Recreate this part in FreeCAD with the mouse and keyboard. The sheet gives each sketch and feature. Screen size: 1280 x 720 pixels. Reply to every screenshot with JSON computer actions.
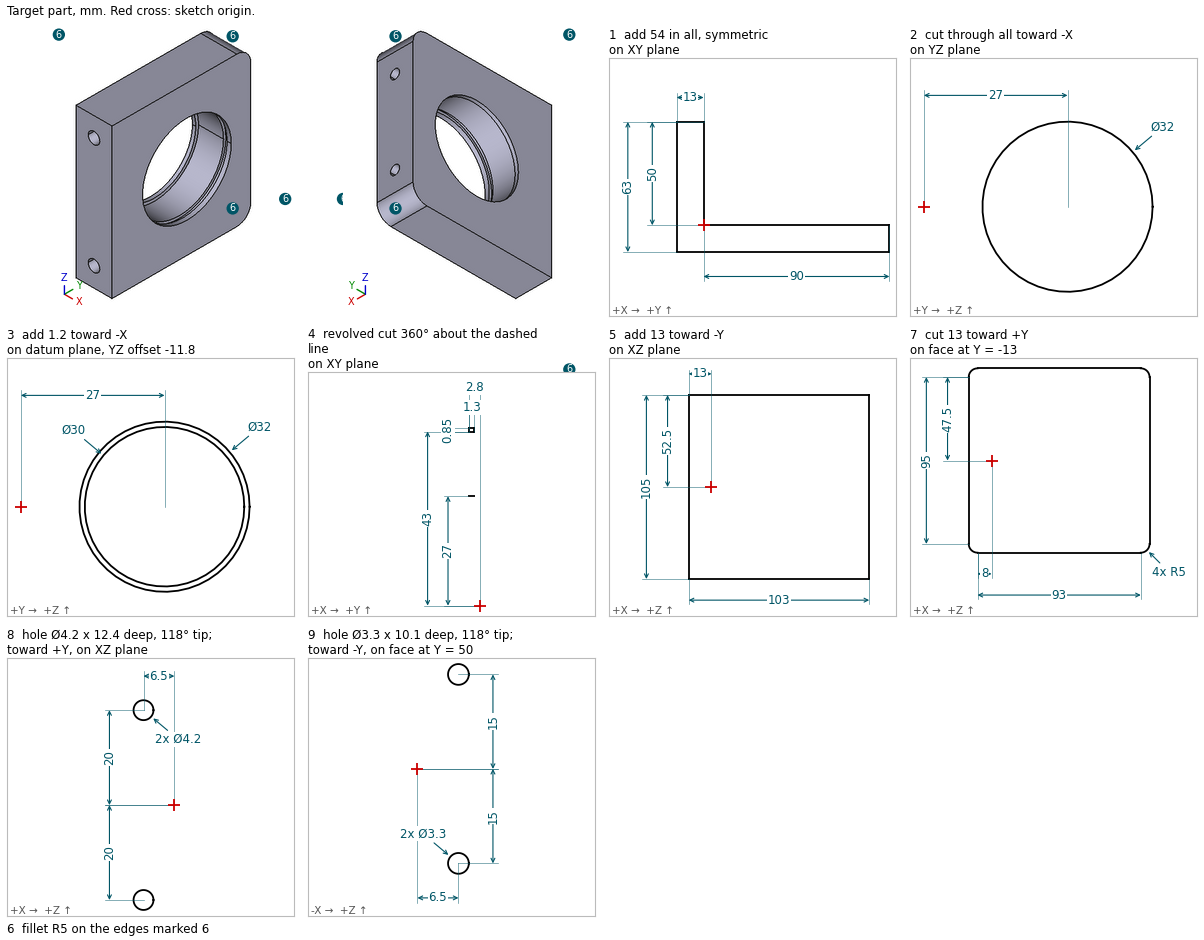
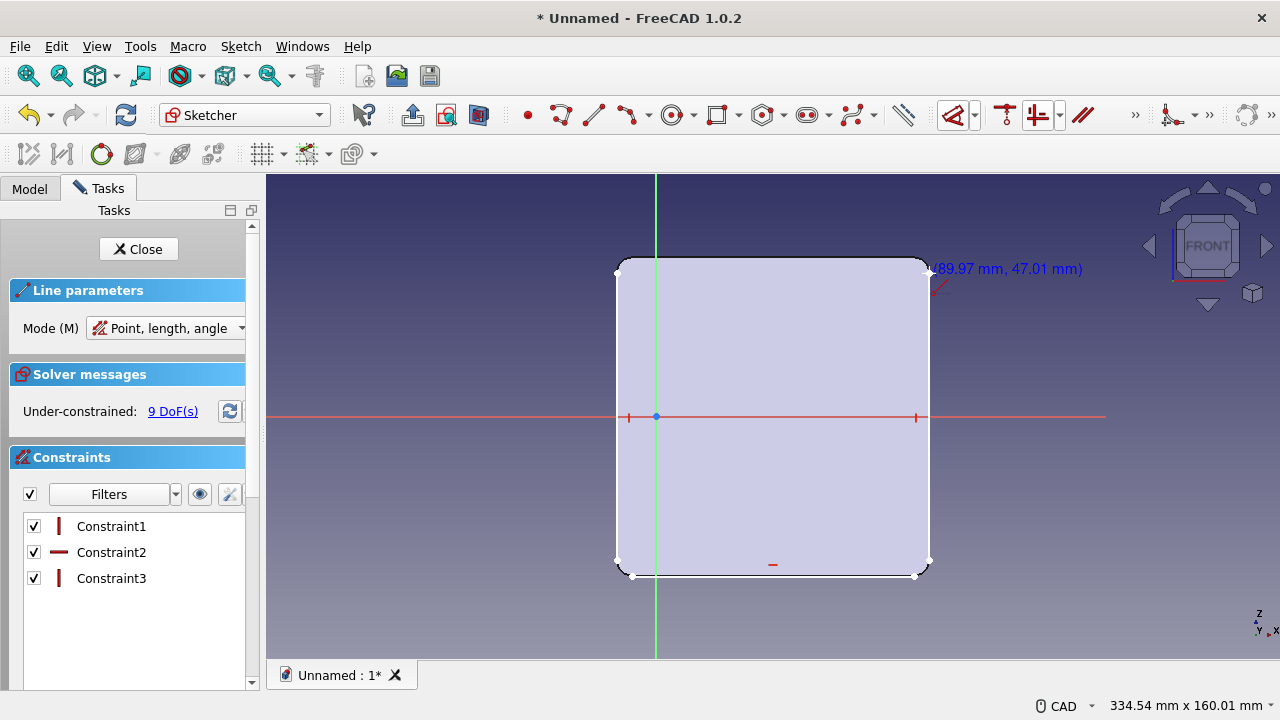
{"action": "left_click", "coordinate": [914, 257]}
{"action": "left_click", "coordinate": [632, 257]}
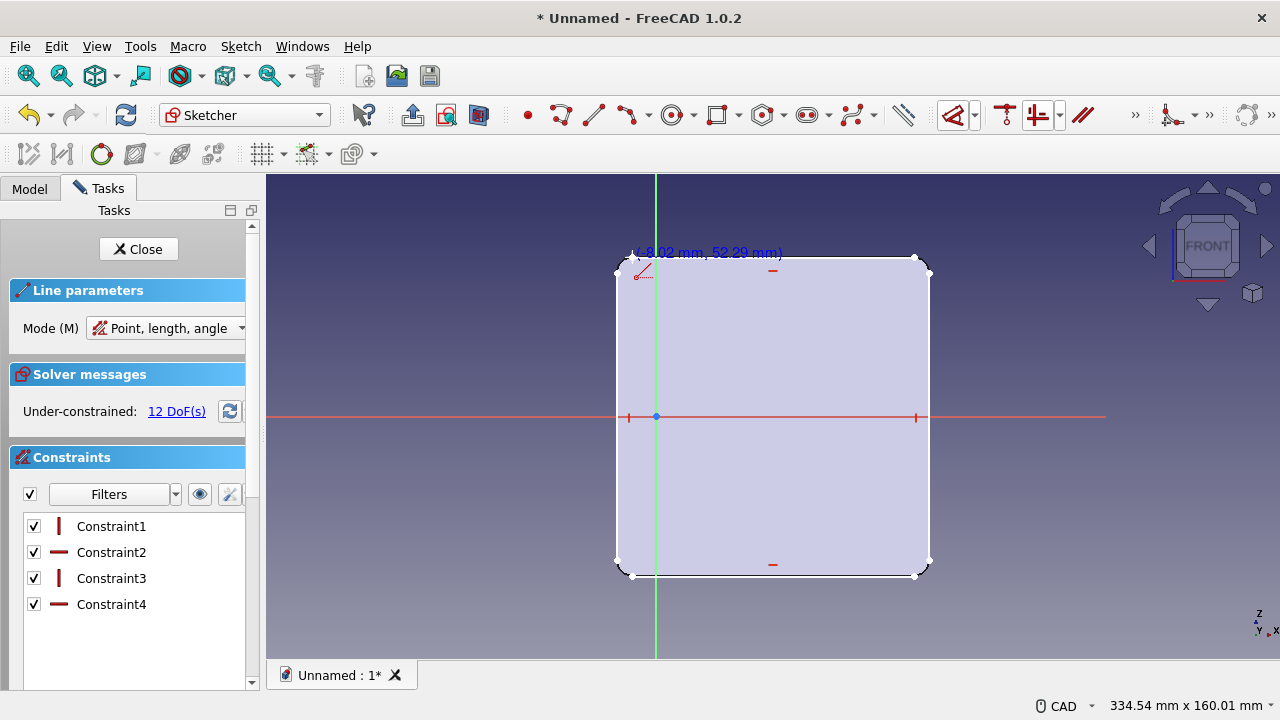
{"action": "left_click", "coordinate": [626, 116]}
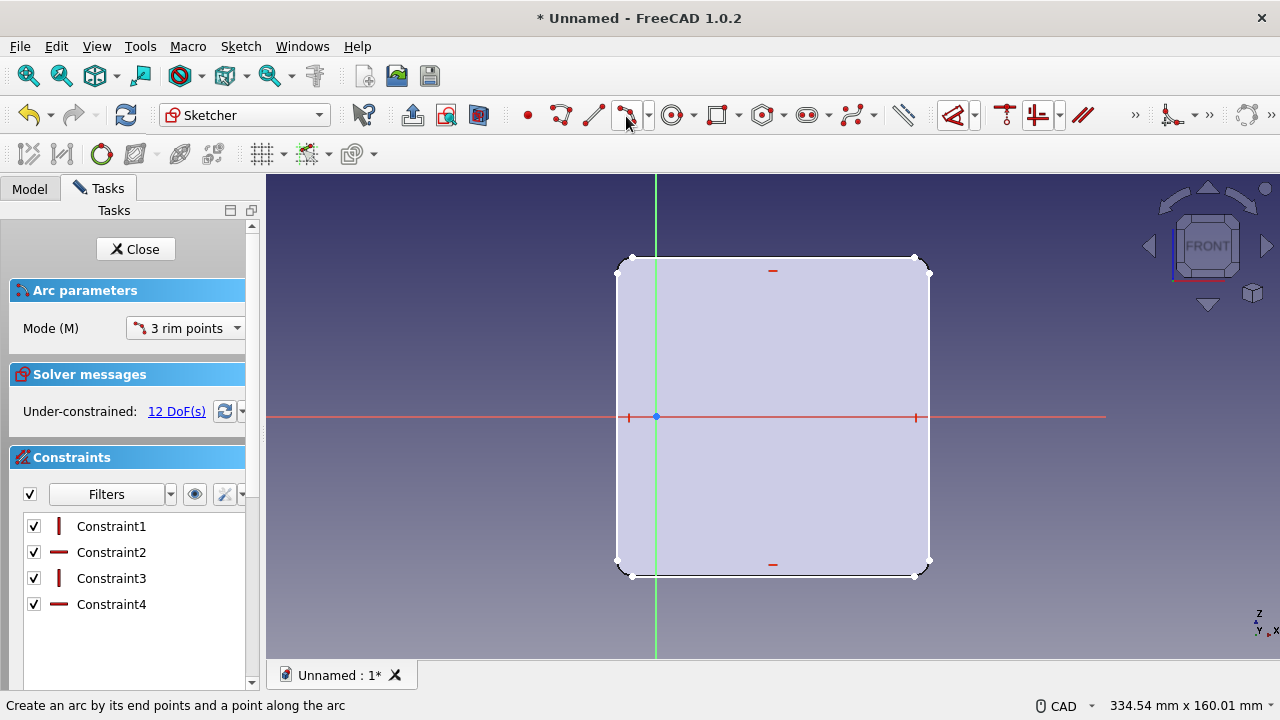
{"action": "left_click", "coordinate": [617, 561]}
{"action": "left_click", "coordinate": [632, 577]}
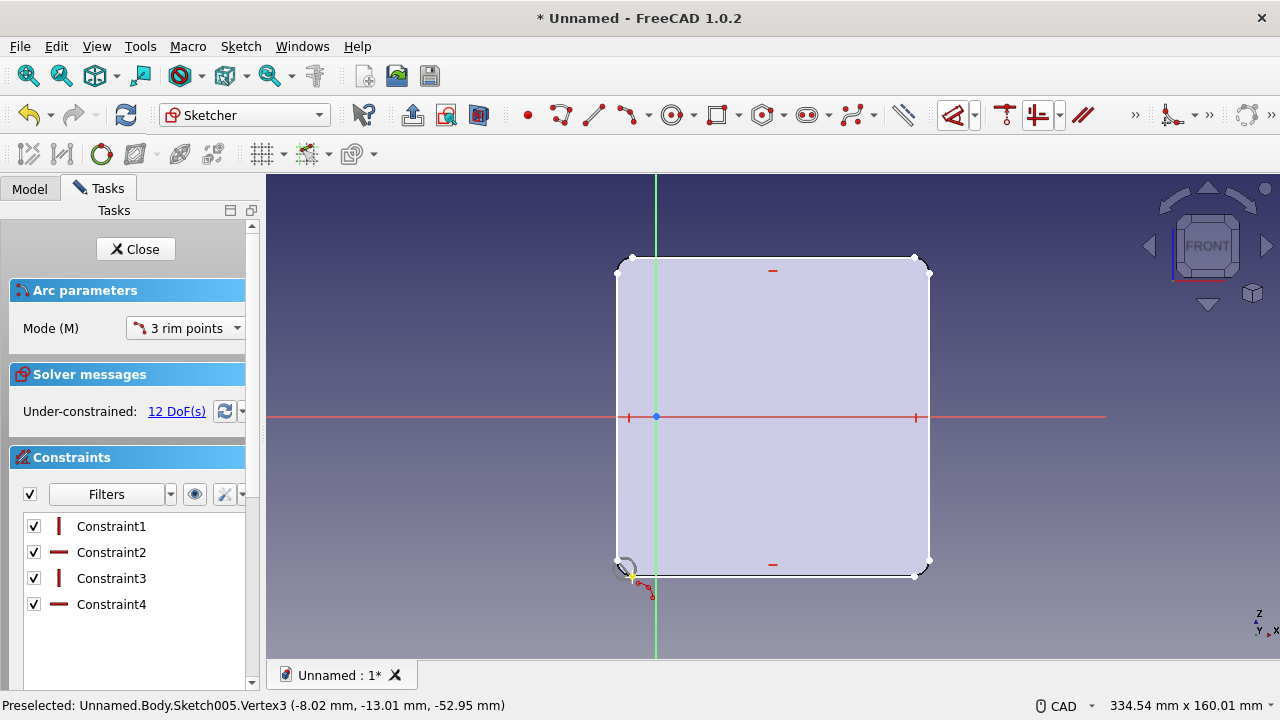
{"action": "scroll", "coordinate": [621, 571], "scroll_direction": "up", "scroll_amount": 7}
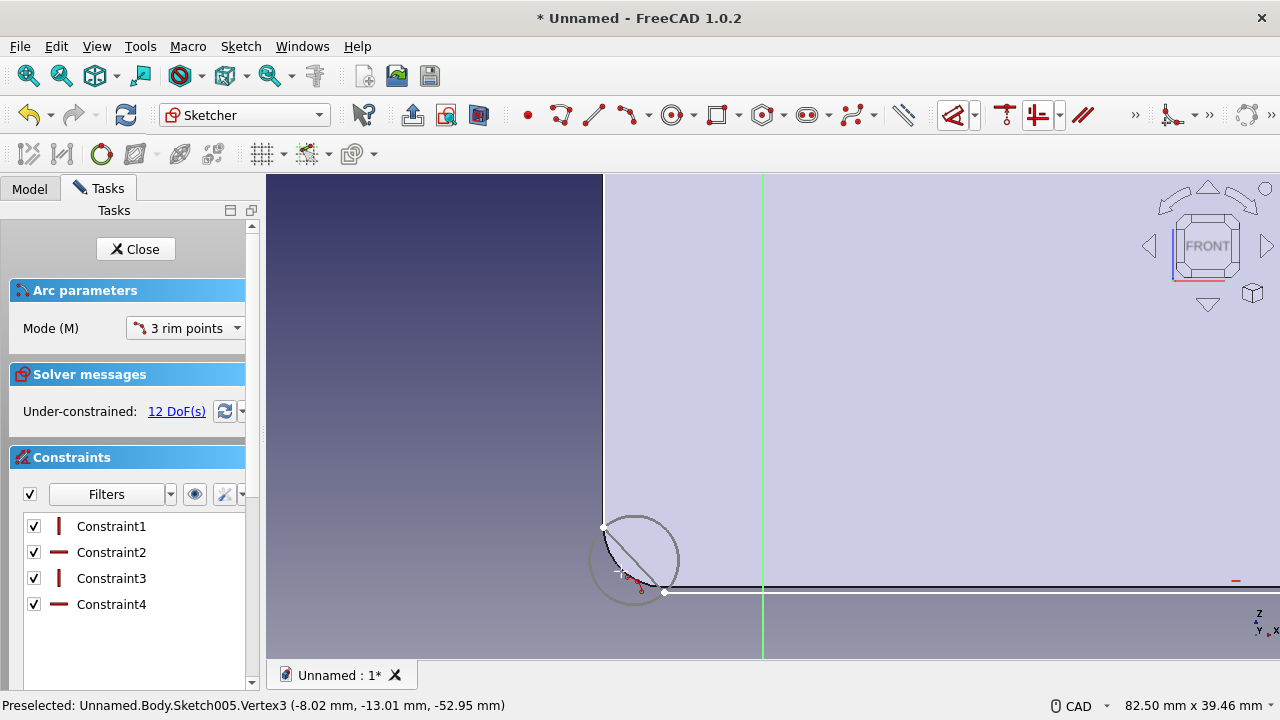
{"action": "left_click", "coordinate": [621, 569]}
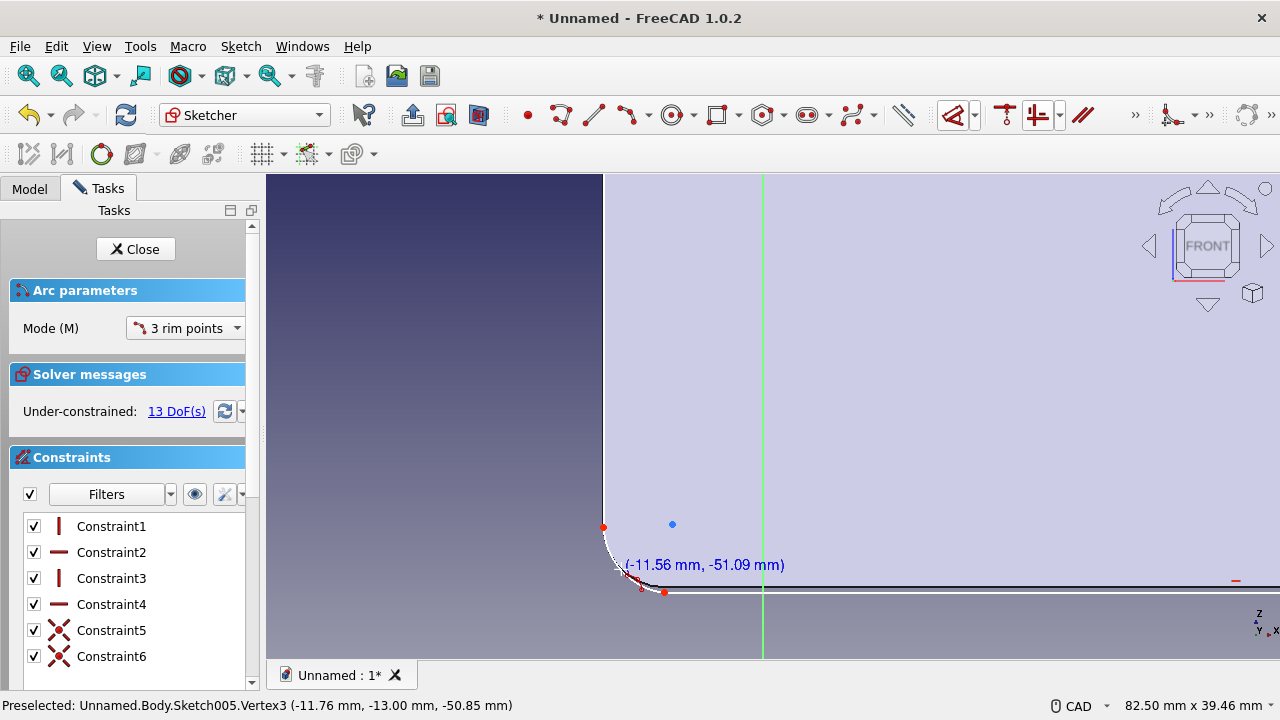
{"action": "scroll", "coordinate": [530, 572], "scroll_direction": "down", "scroll_amount": 7}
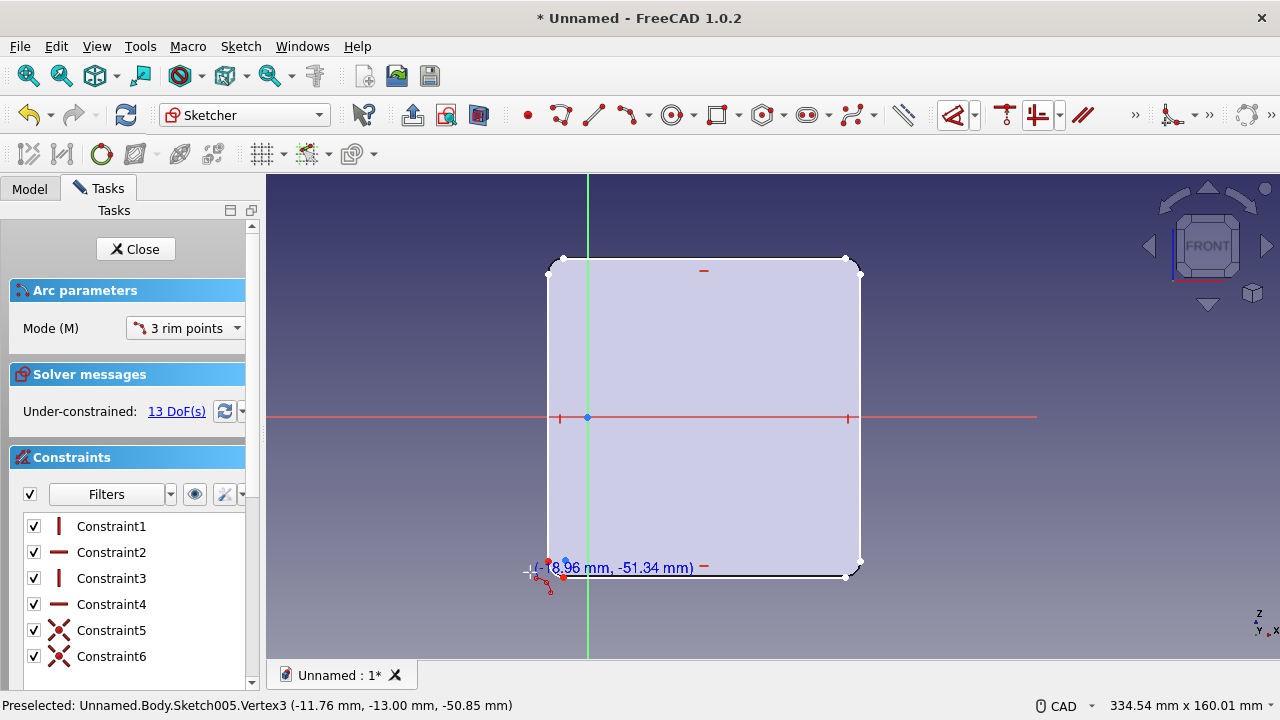
{"action": "left_click", "coordinate": [845, 578]}
{"action": "left_click", "coordinate": [860, 562]}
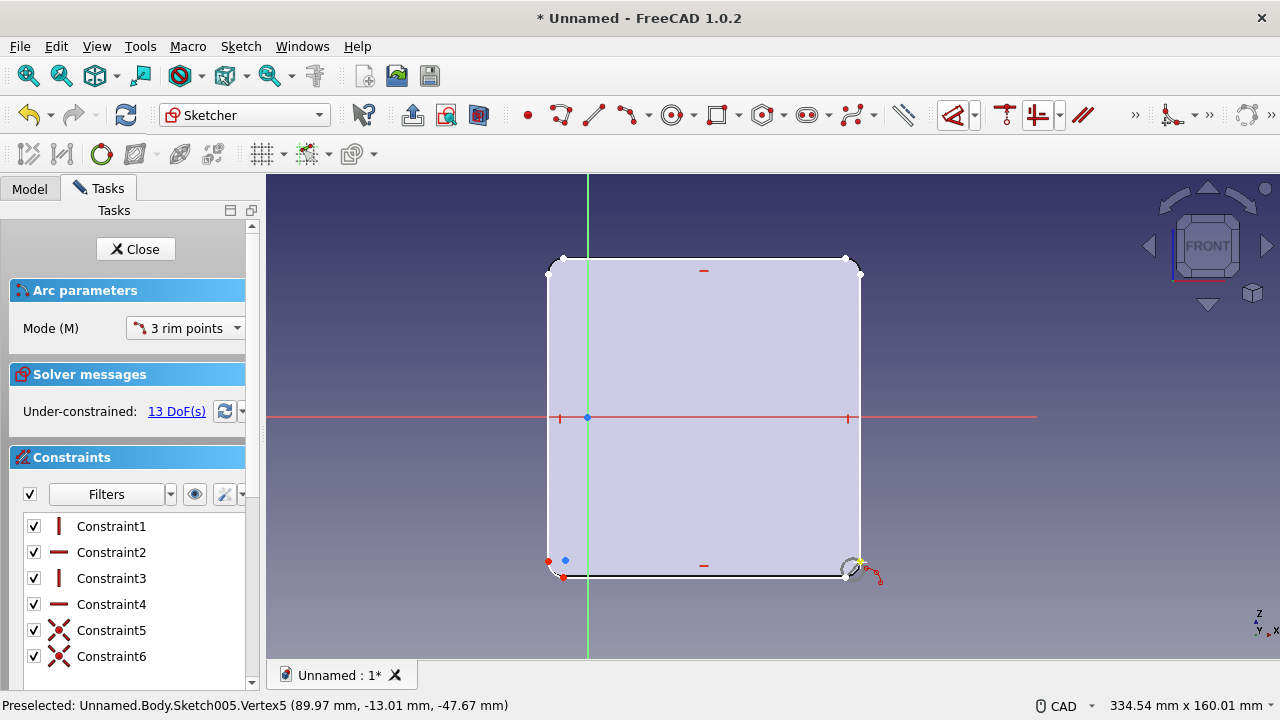
{"action": "scroll", "coordinate": [856, 572], "scroll_direction": "up", "scroll_amount": 7}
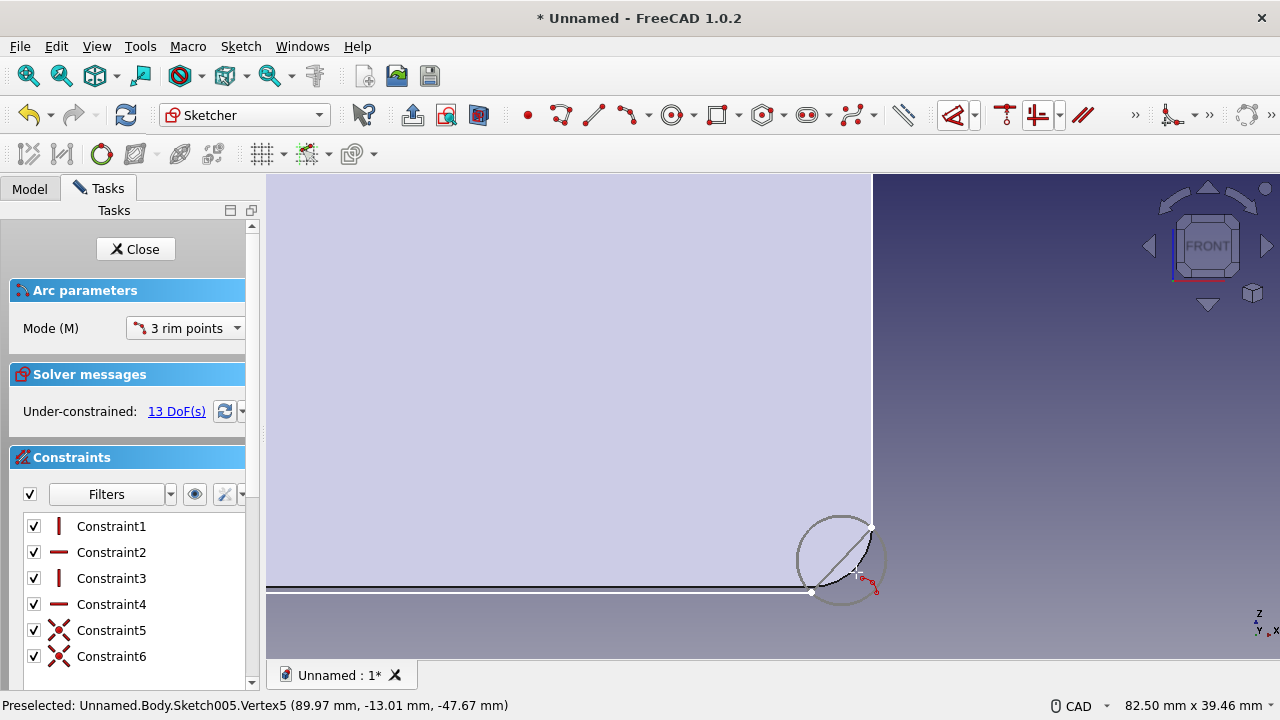
{"action": "left_click", "coordinate": [854, 569]}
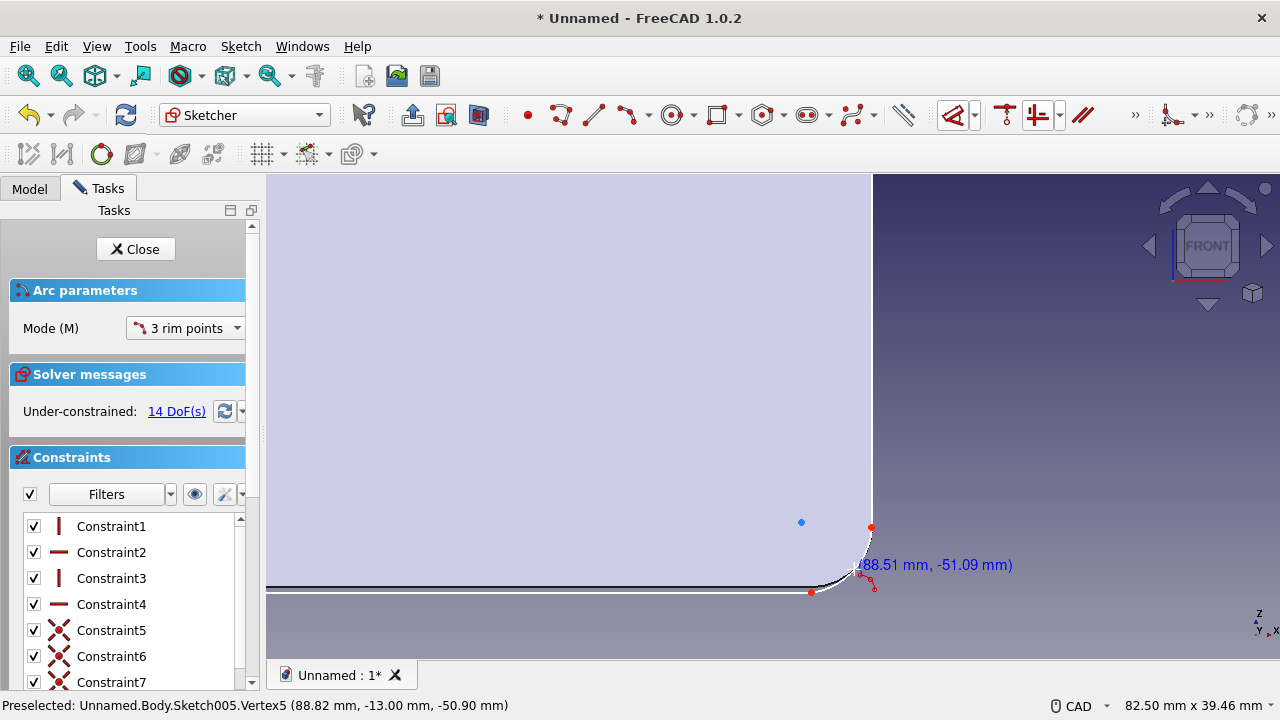
{"action": "scroll", "coordinate": [857, 572], "scroll_direction": "down", "scroll_amount": 7}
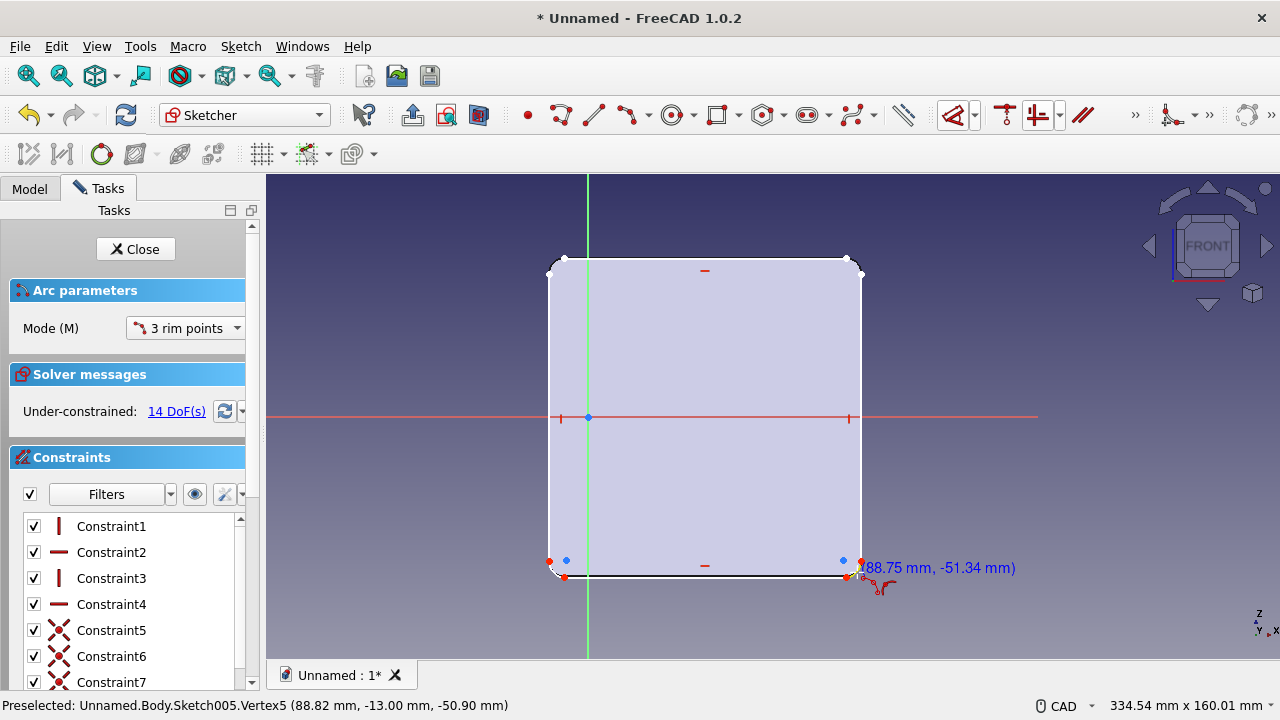
{"action": "left_click", "coordinate": [861, 275]}
{"action": "left_click", "coordinate": [846, 259]}